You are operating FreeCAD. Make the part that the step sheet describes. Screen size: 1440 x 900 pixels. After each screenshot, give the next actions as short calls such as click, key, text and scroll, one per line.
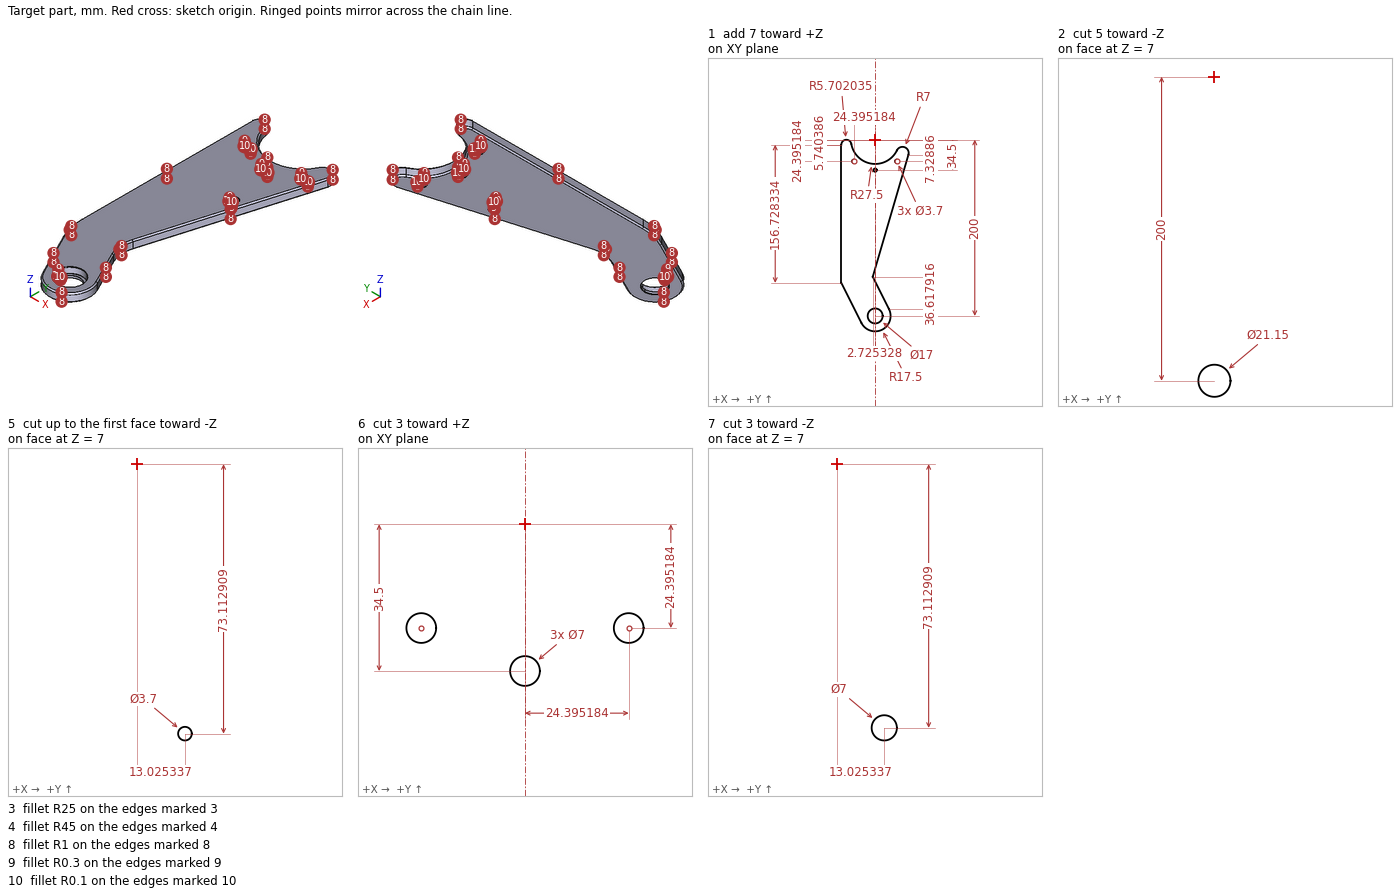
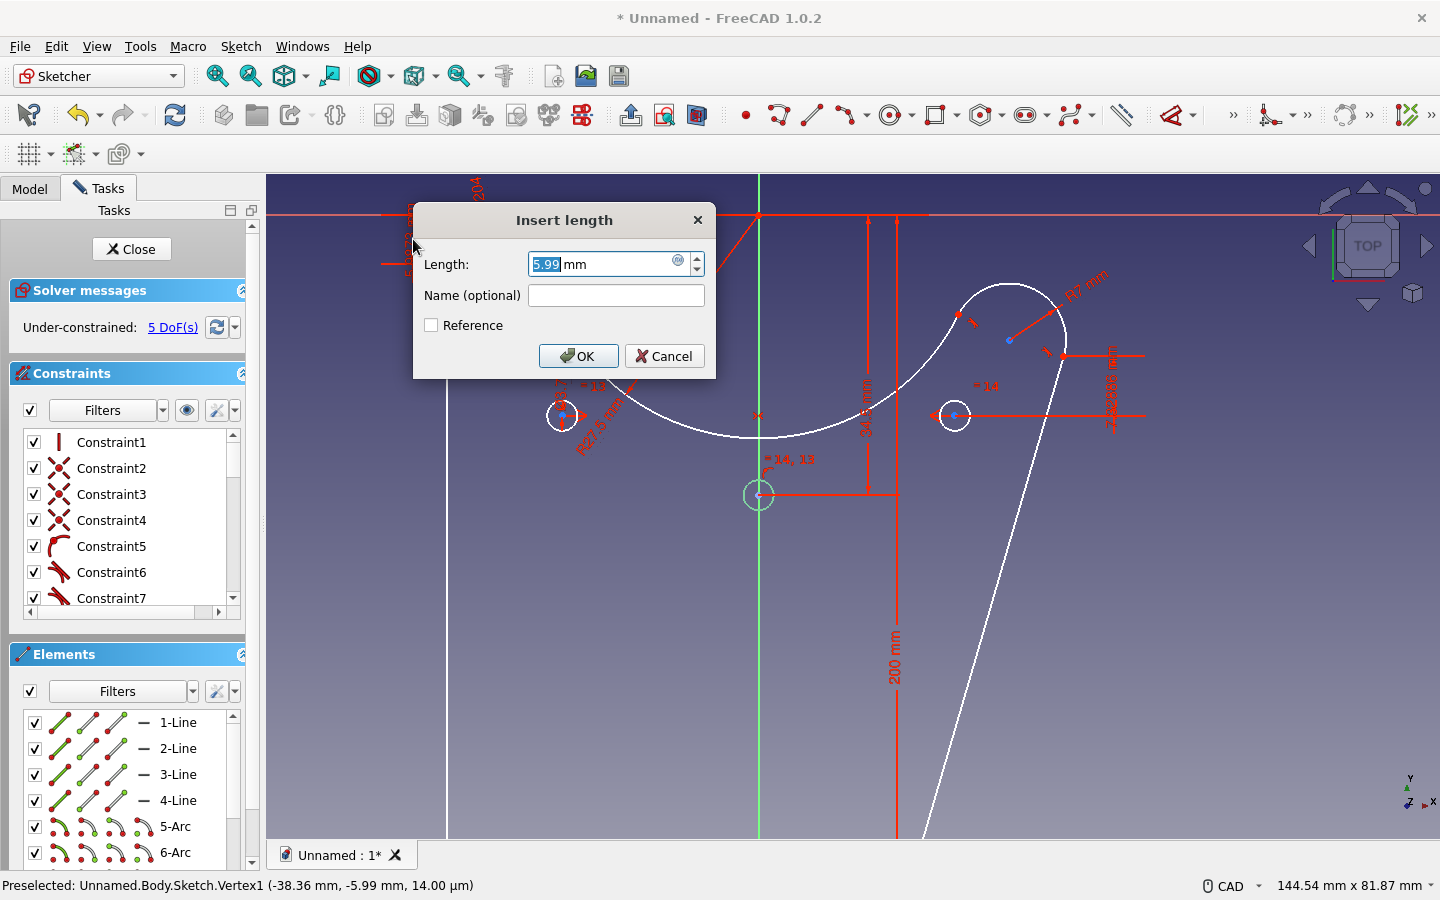
text(5.740386)
key(Return)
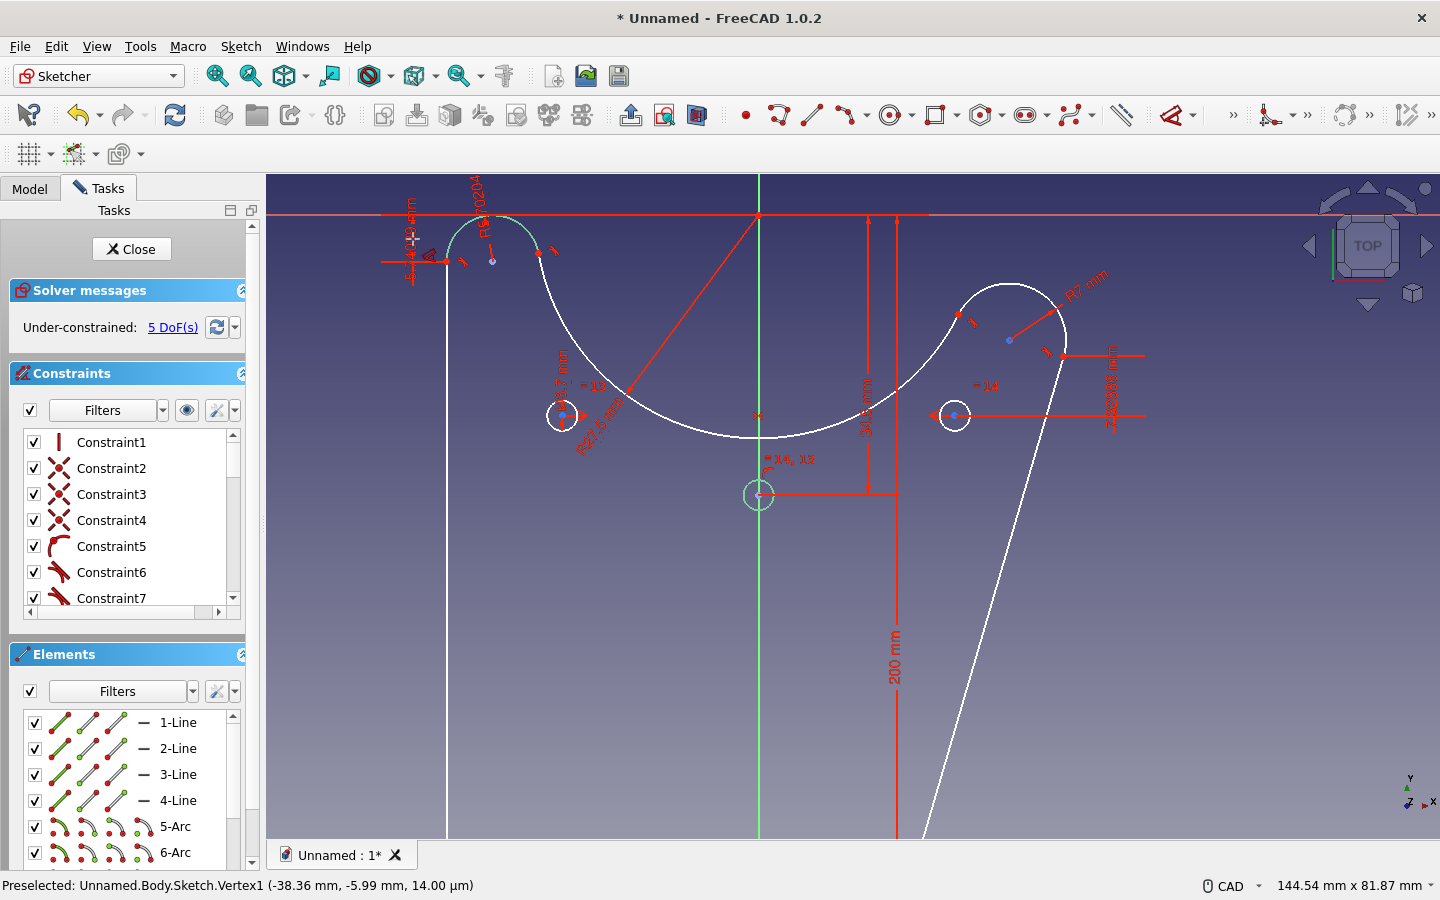
scroll(794, 315, down, 7)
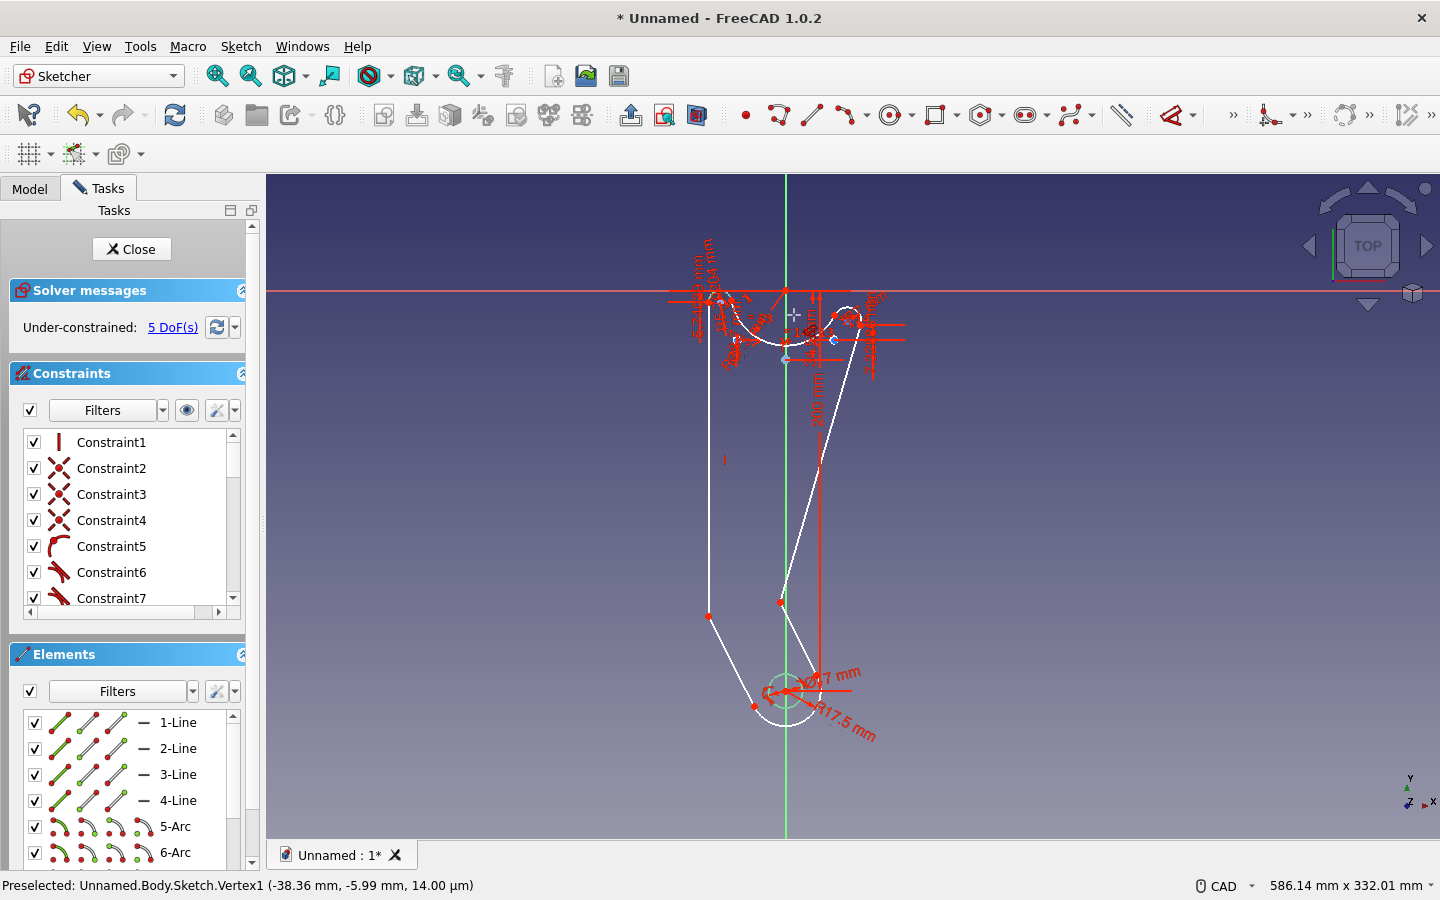
scroll(780, 602, up, 10)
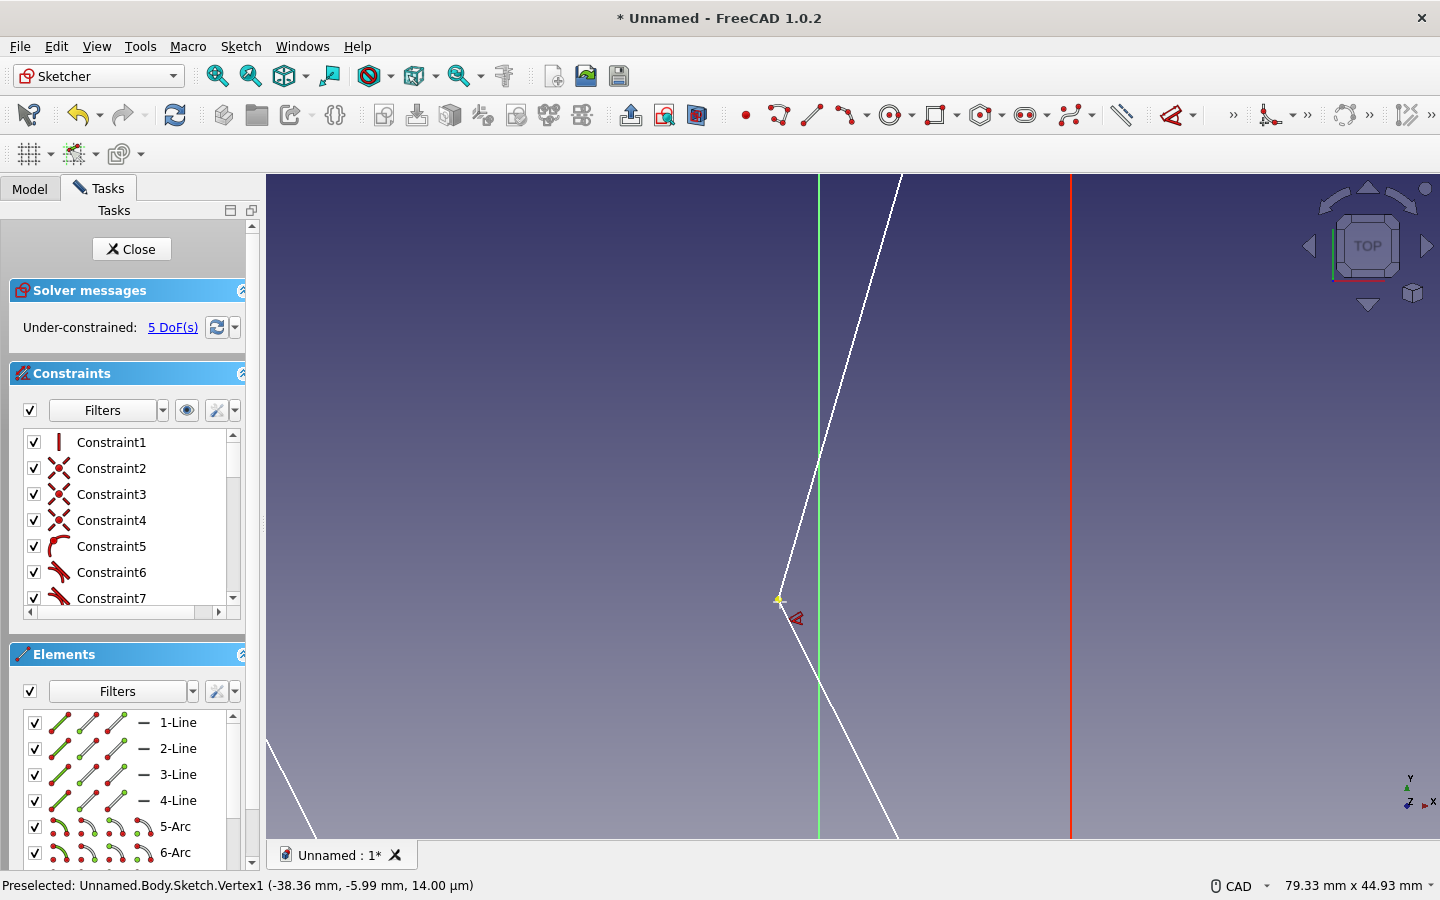
click(778, 599)
click(789, 657)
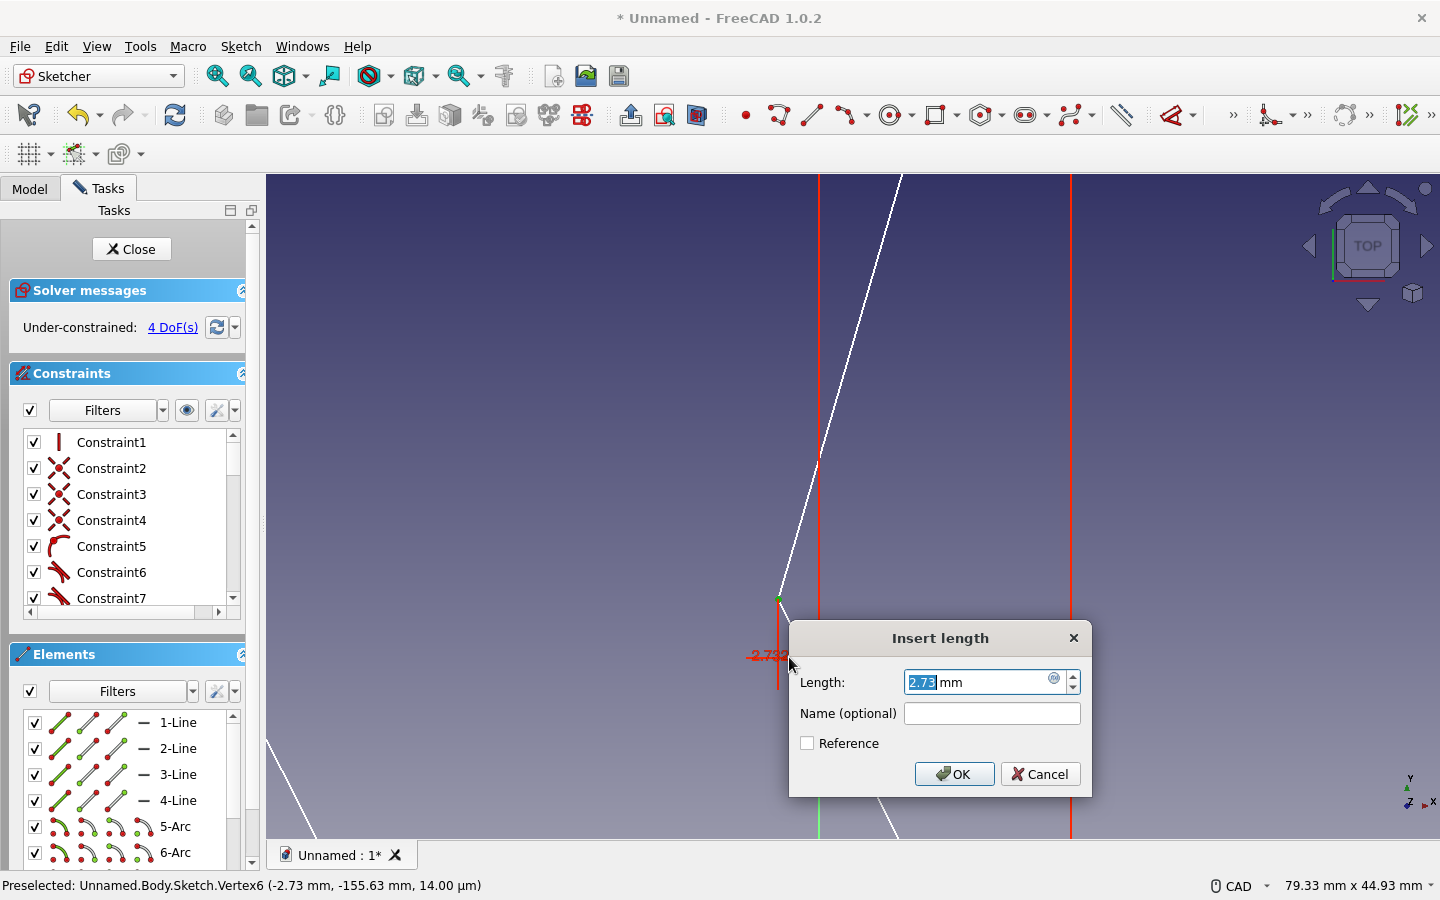
text(2.725328)
key(Return)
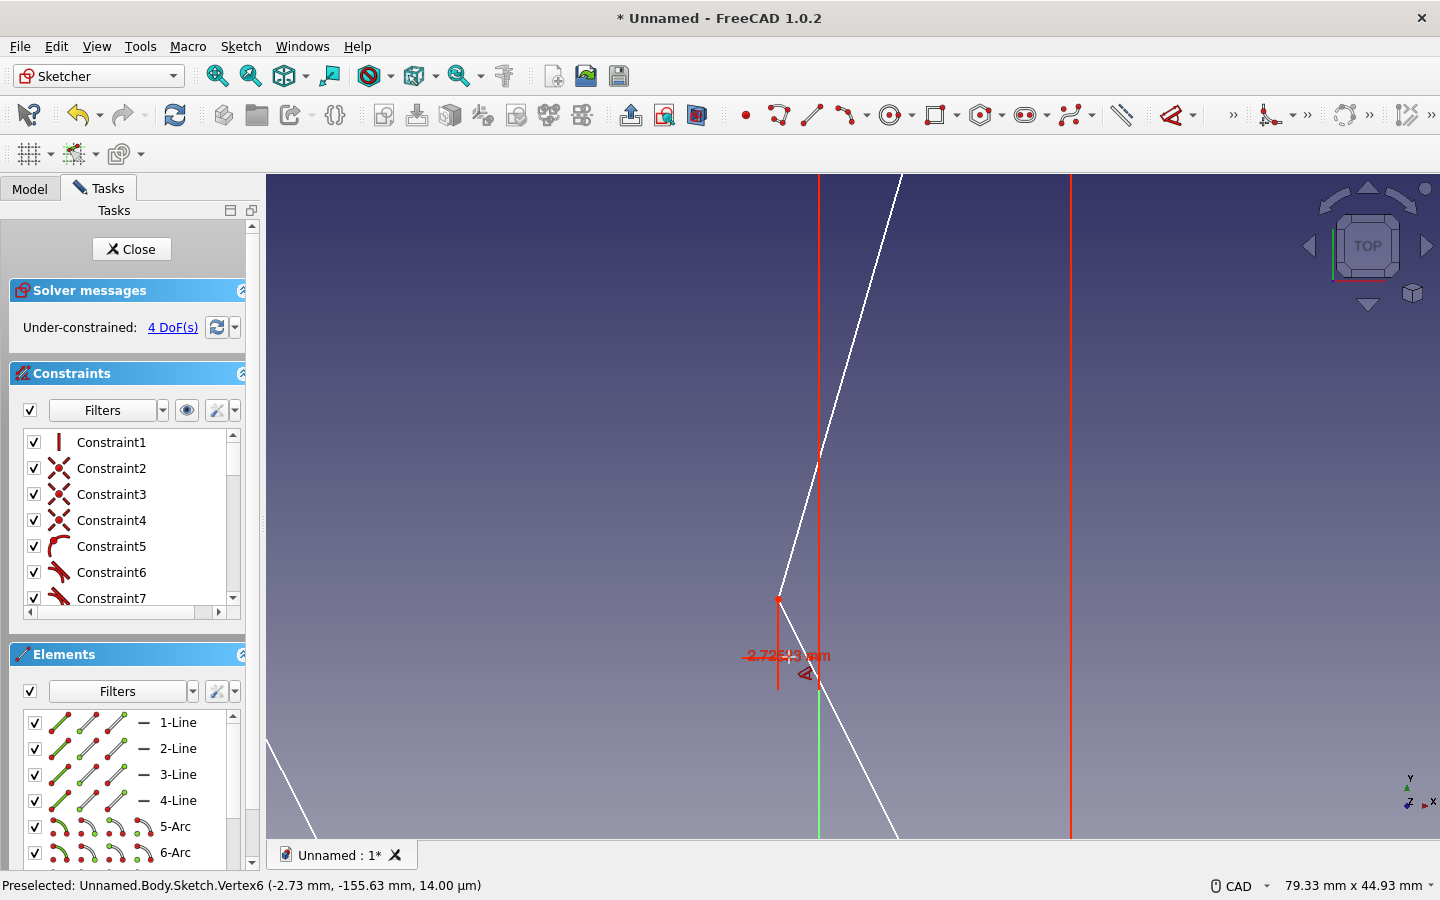
scroll(780, 603, down, 10)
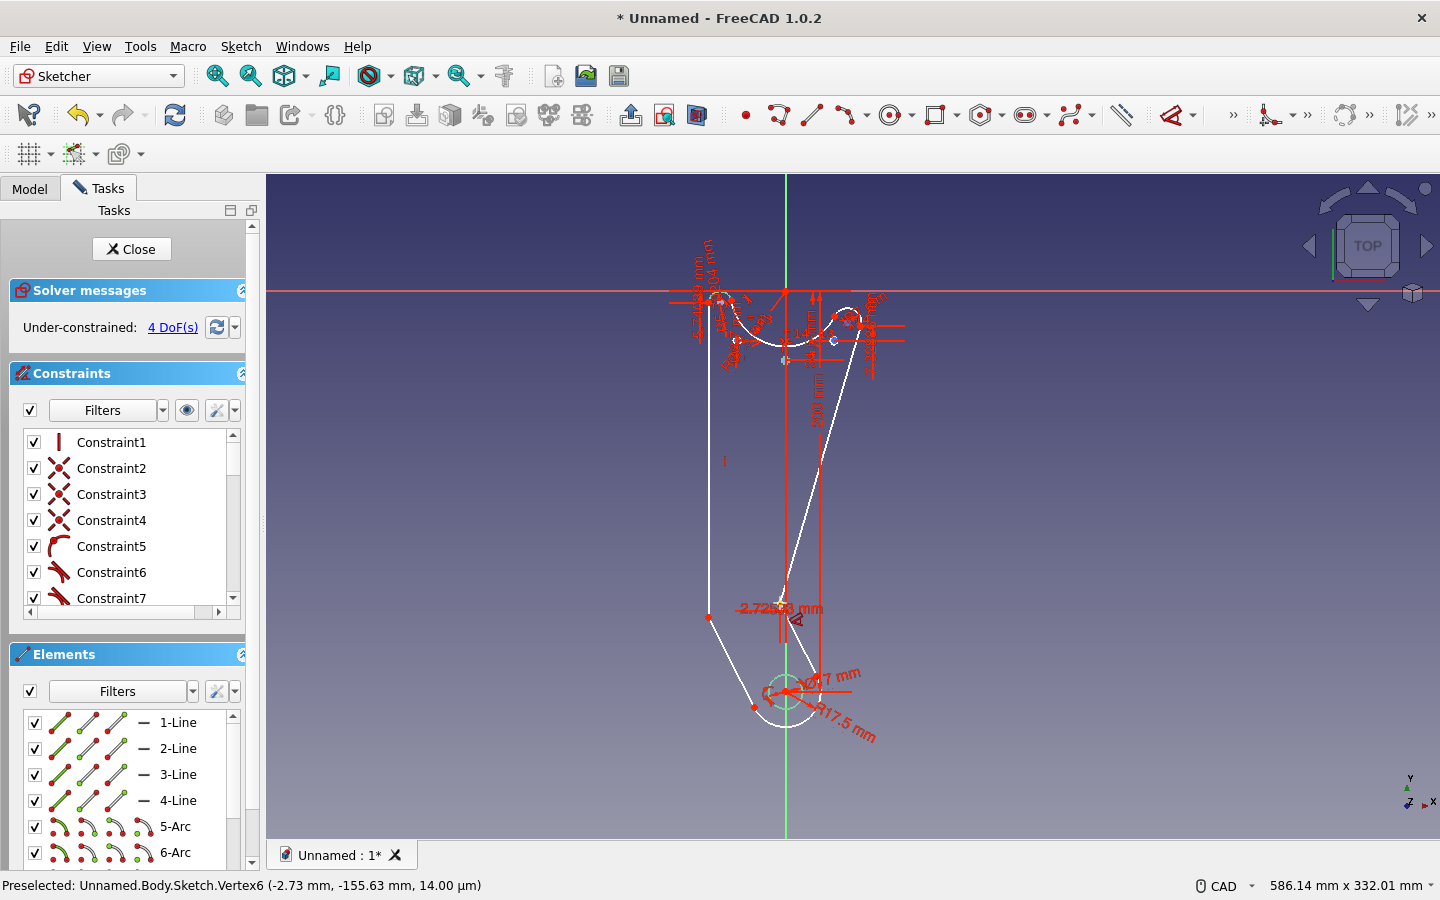
click(737, 341)
click(761, 257)